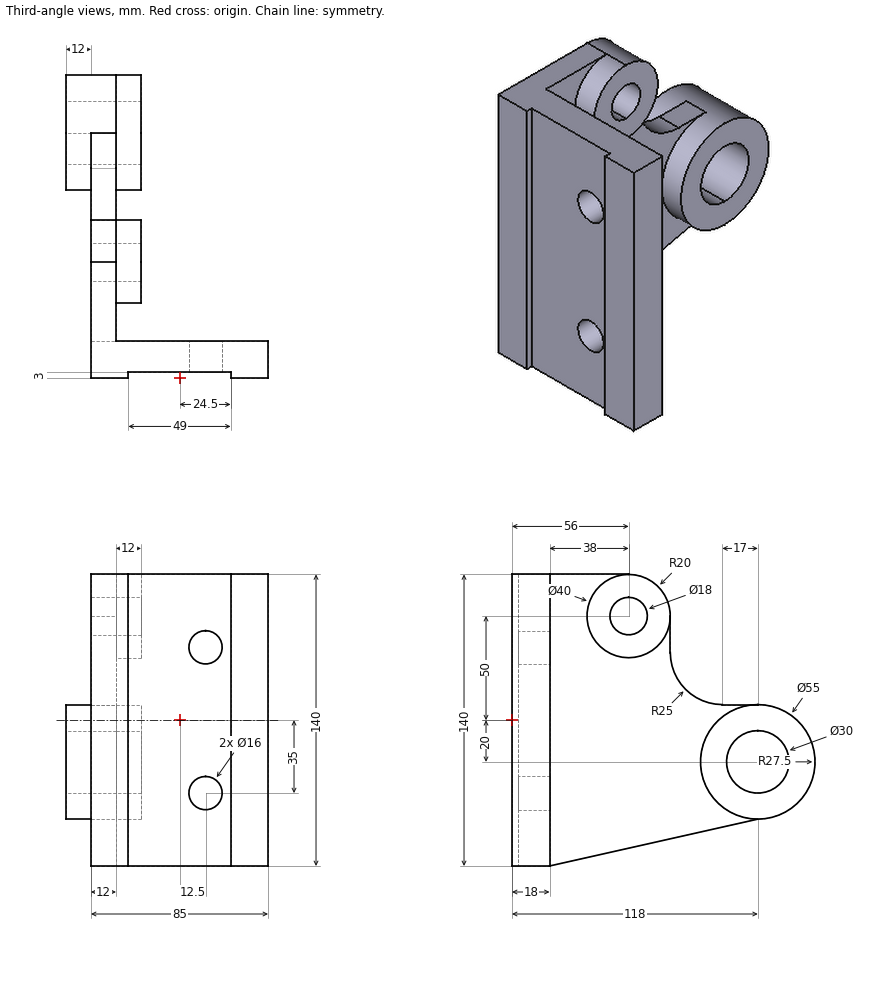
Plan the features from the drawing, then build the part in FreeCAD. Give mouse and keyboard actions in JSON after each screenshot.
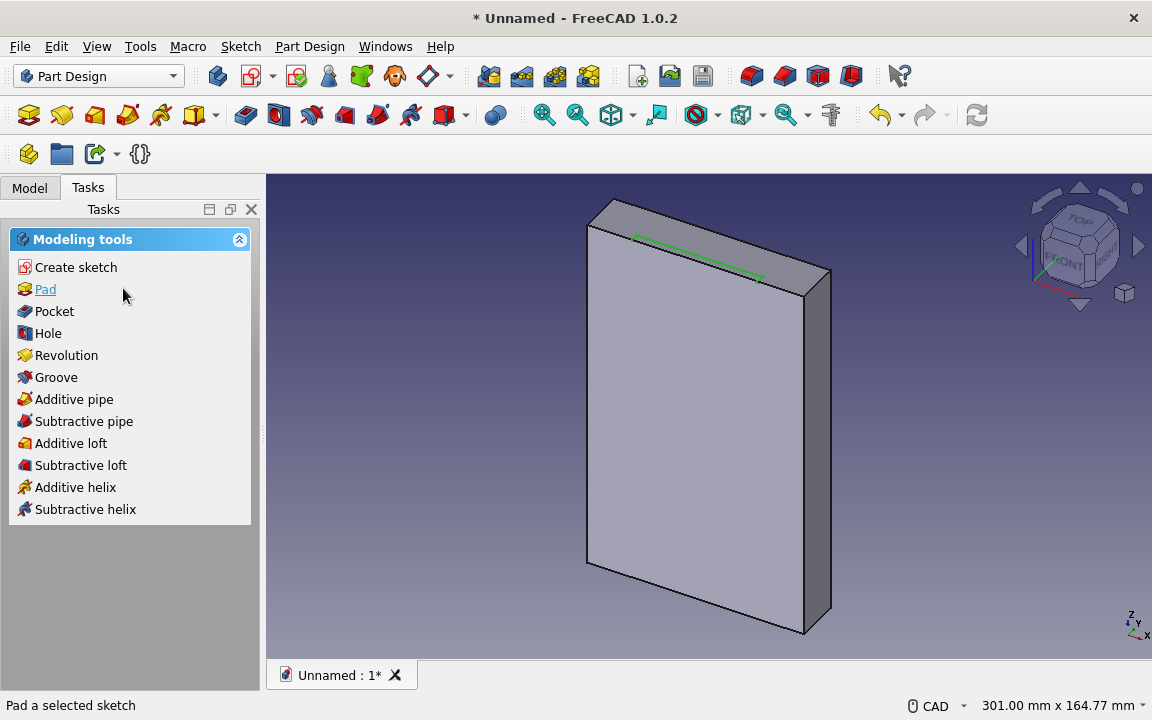
{"action": "left_click", "coordinate": [246, 116]}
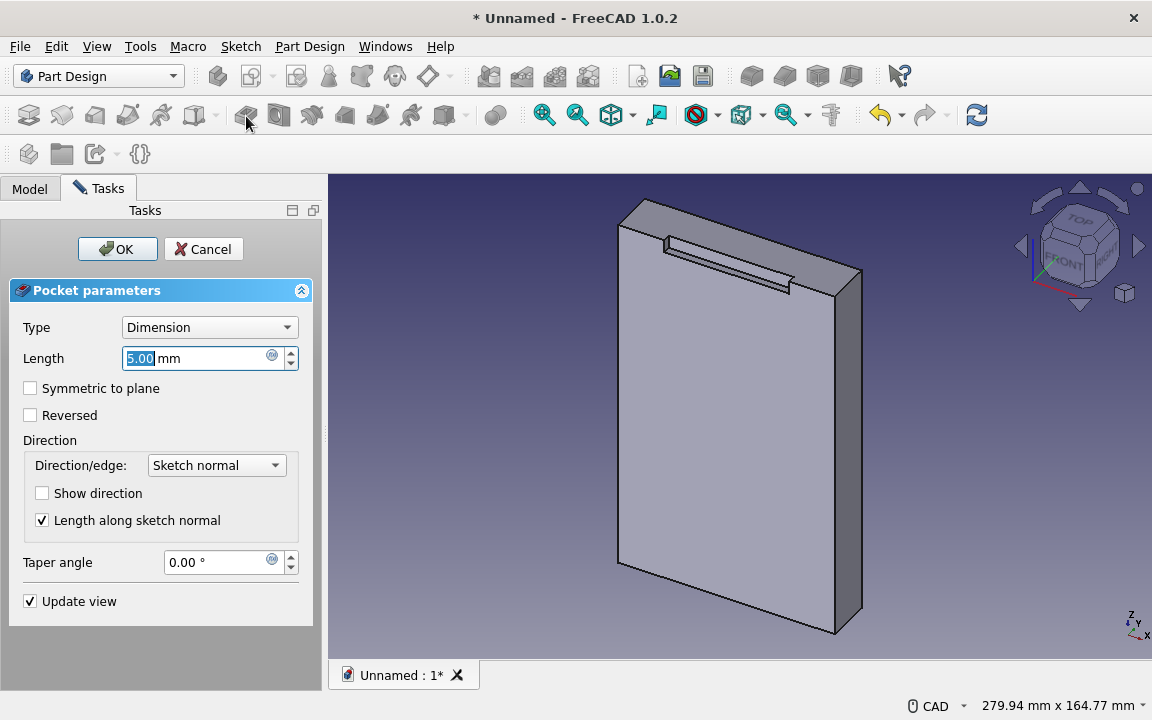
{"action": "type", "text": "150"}
{"action": "key", "text": "Tab"}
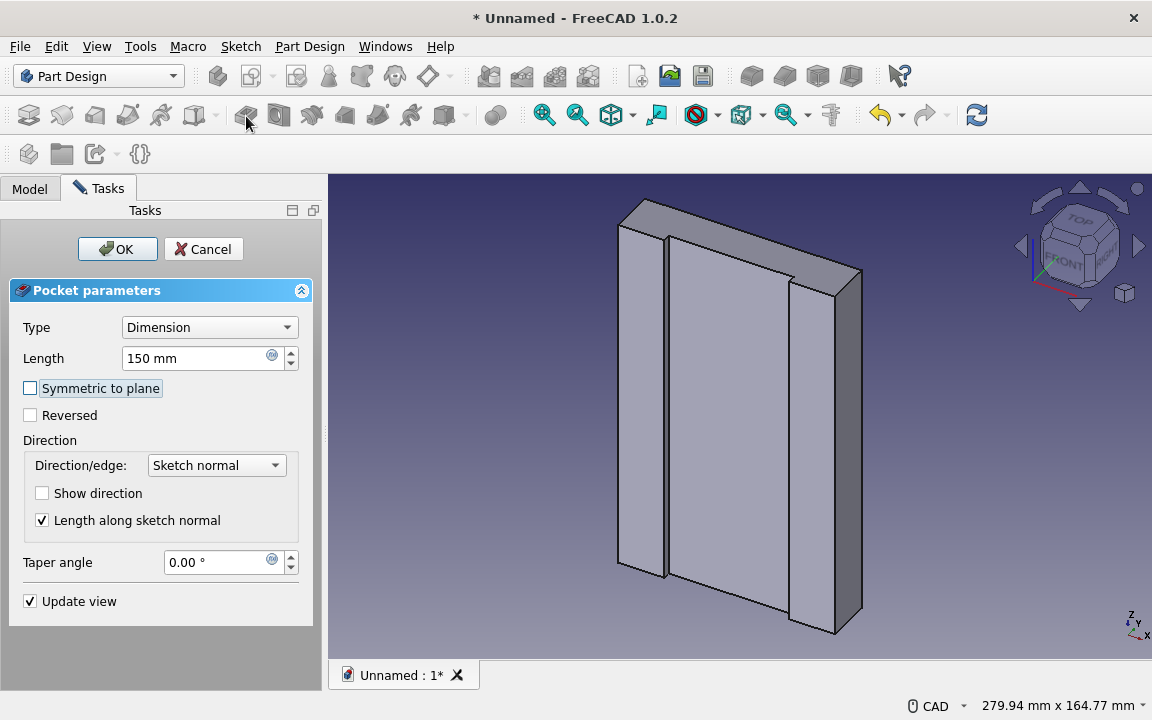
{"action": "left_click", "coordinate": [118, 249]}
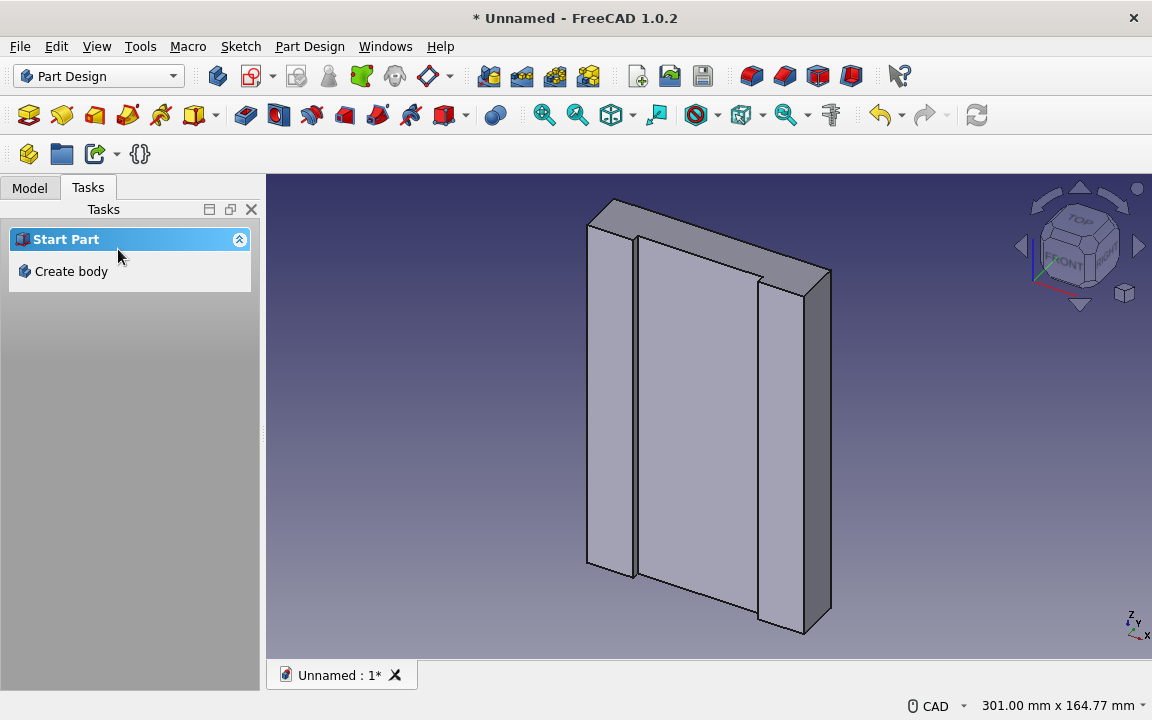
{"action": "key", "text": "6"}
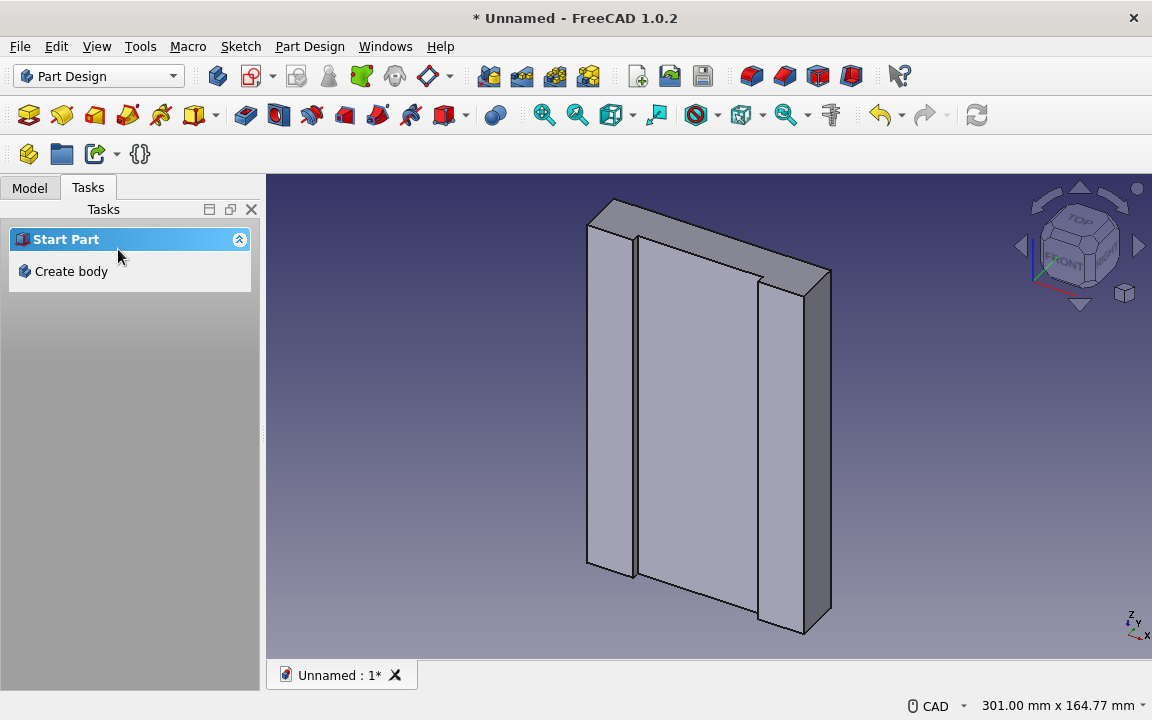
{"action": "left_click", "coordinate": [709, 415]}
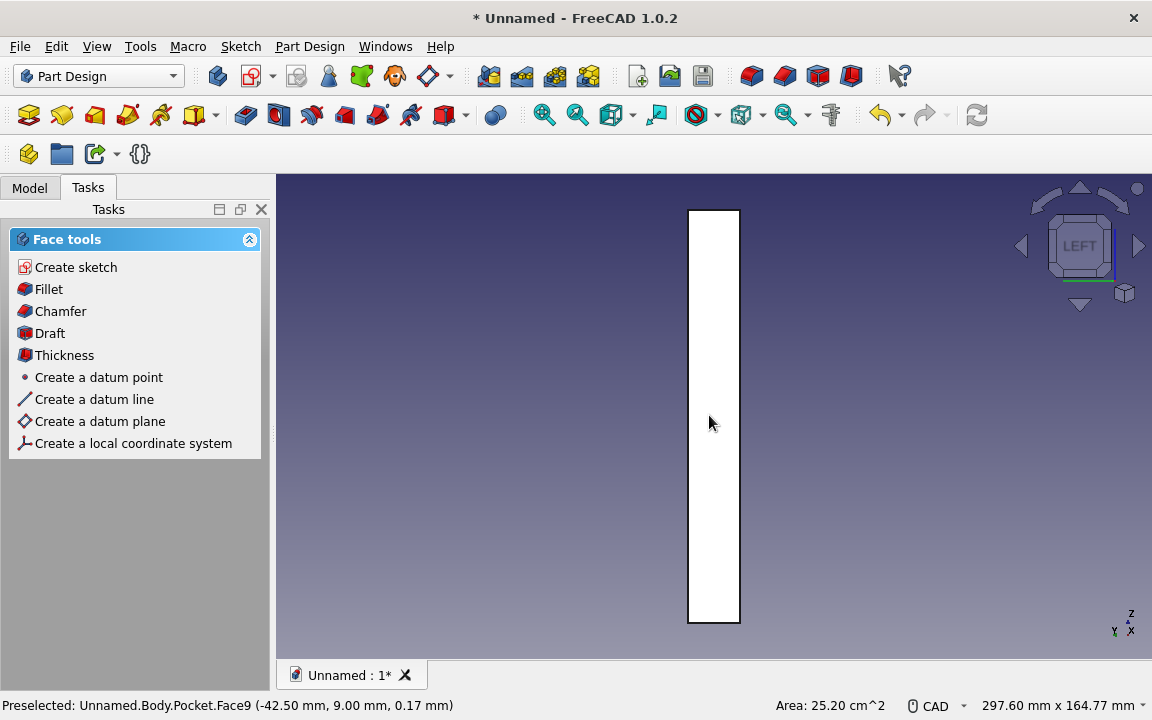
{"action": "left_click", "coordinate": [250, 76]}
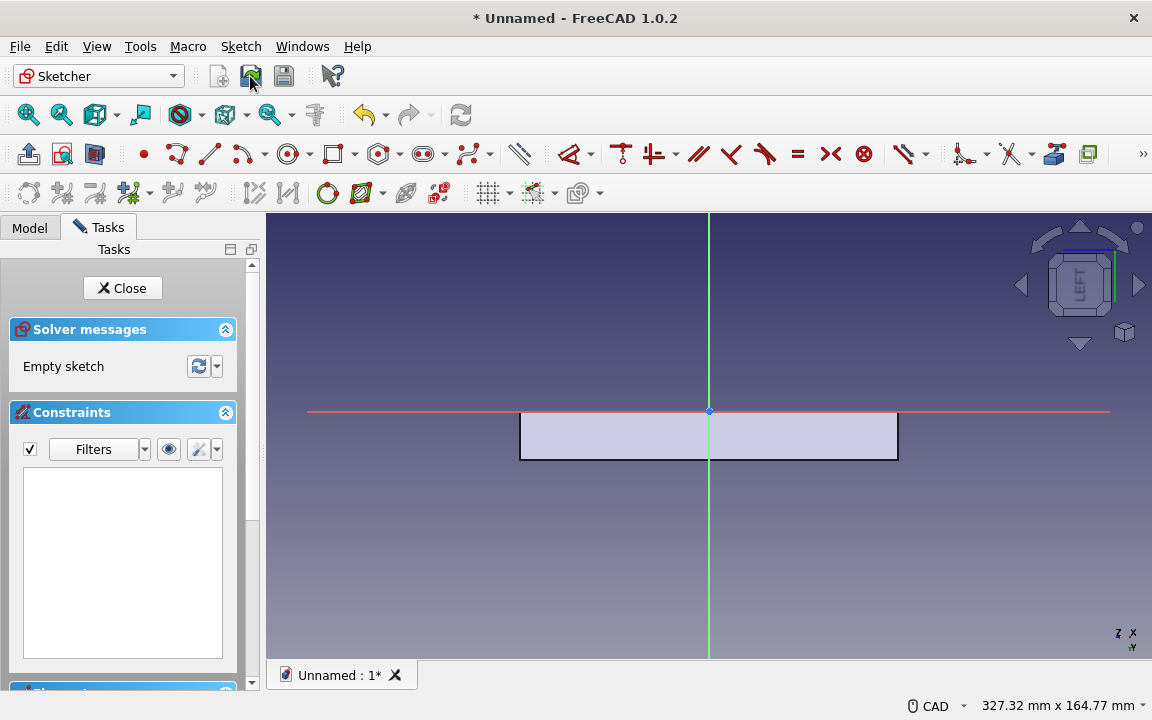
{"action": "scroll", "coordinate": [557, 241], "scroll_direction": "down", "scroll_amount": 3}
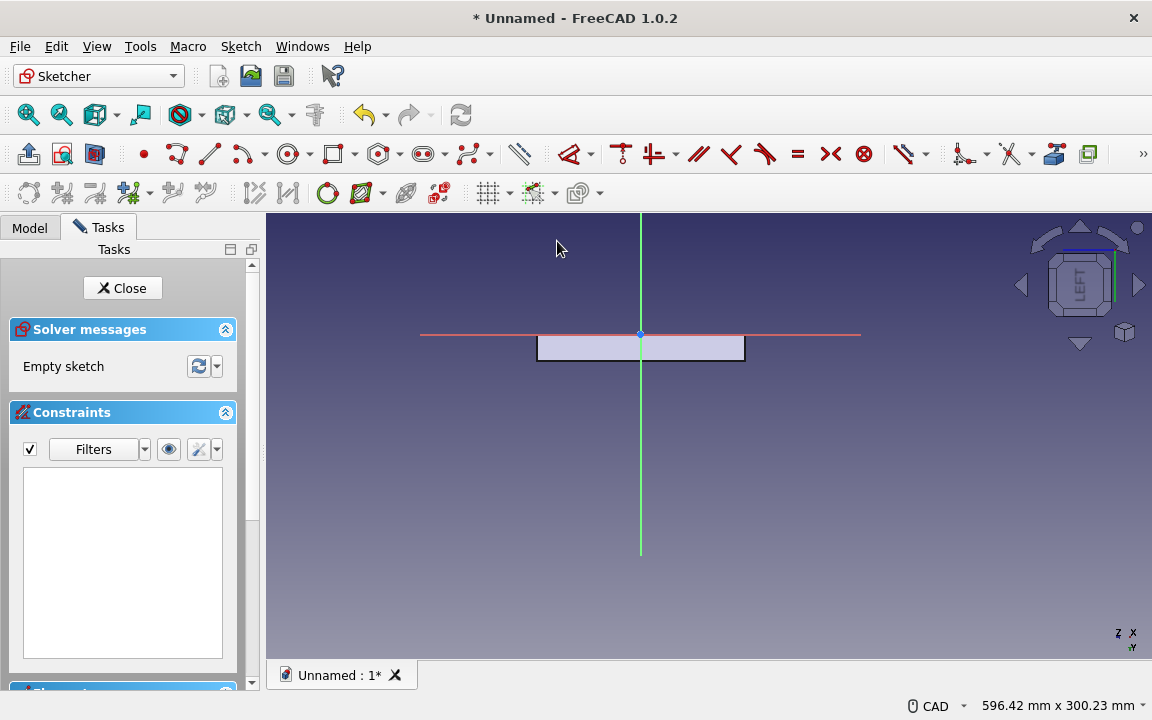
{"action": "left_click", "coordinate": [210, 154]}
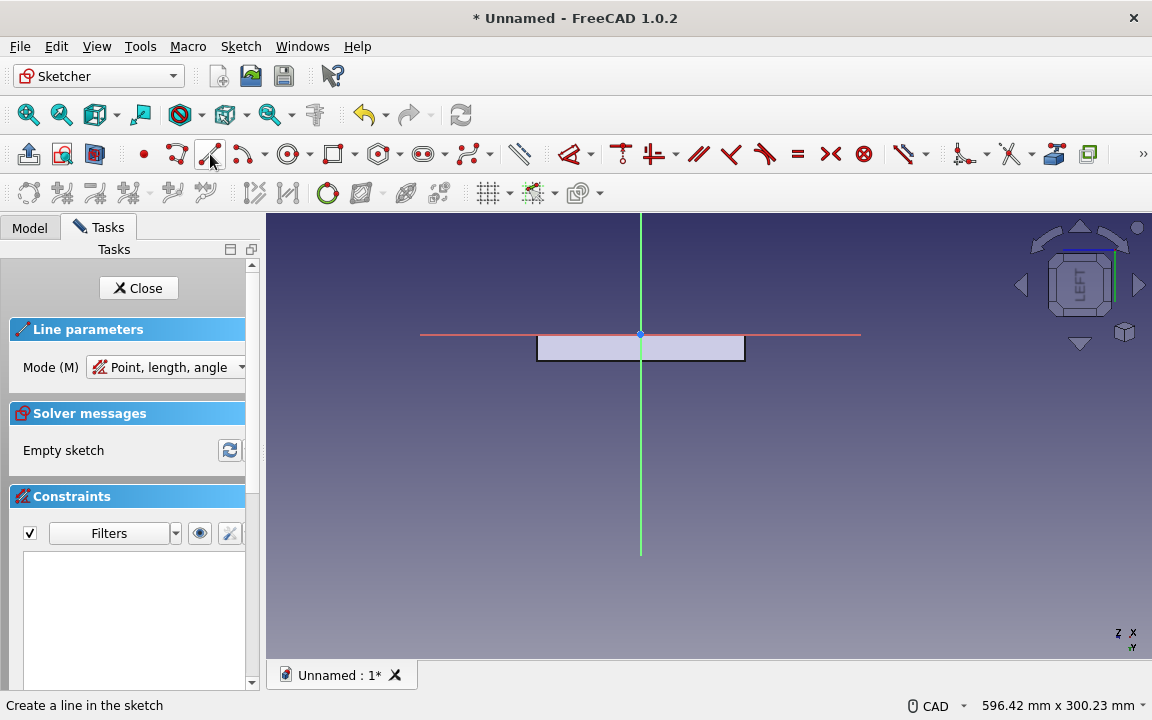
{"action": "left_click", "coordinate": [566, 448]}
{"action": "left_click", "coordinate": [592, 448]}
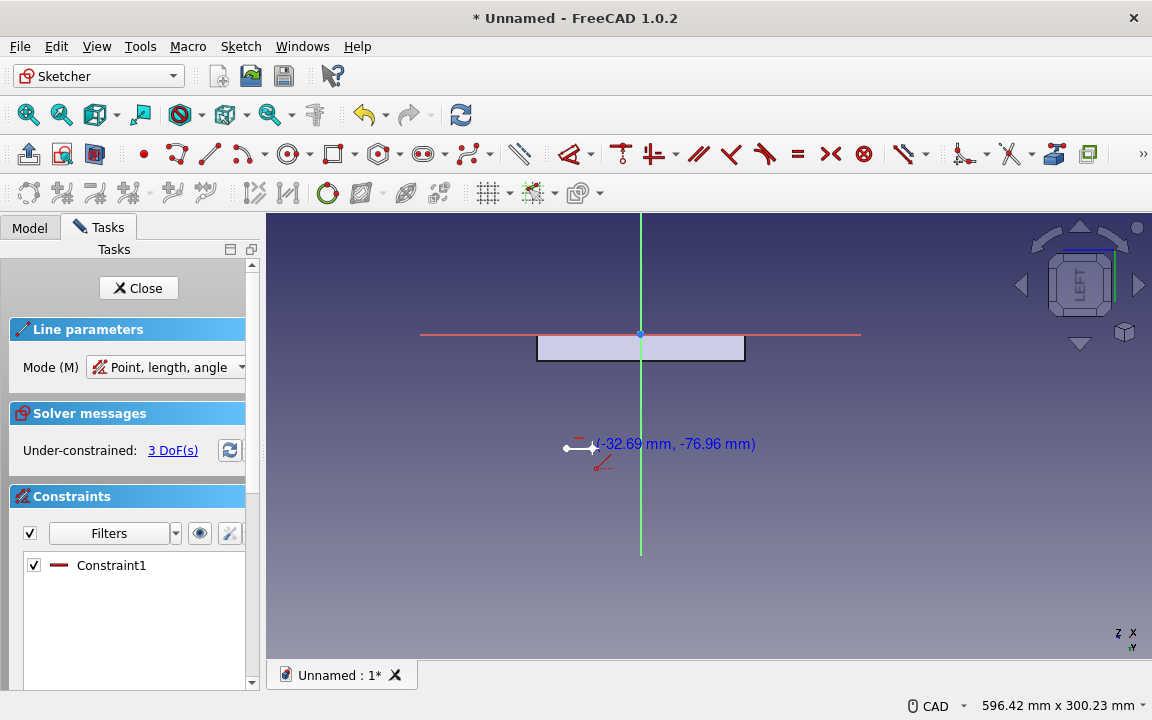
{"action": "scroll", "coordinate": [629, 485], "scroll_direction": "up", "scroll_amount": 2}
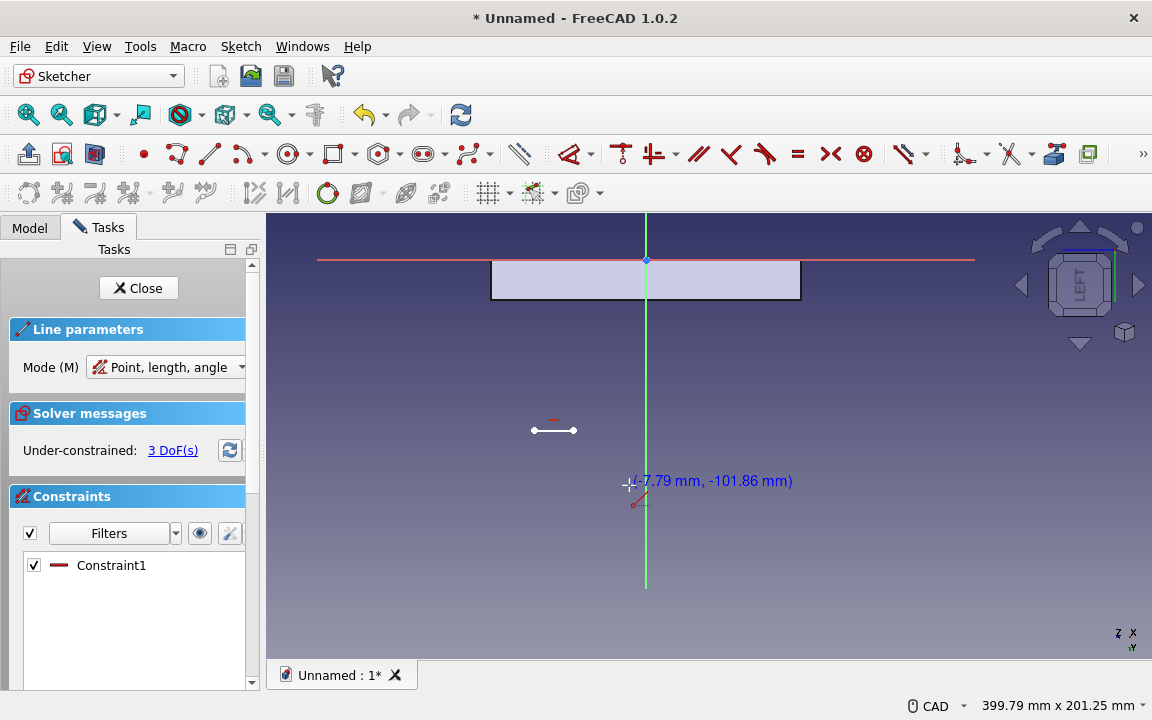
{"action": "left_click", "coordinate": [629, 484]}
{"action": "left_click", "coordinate": [629, 522]}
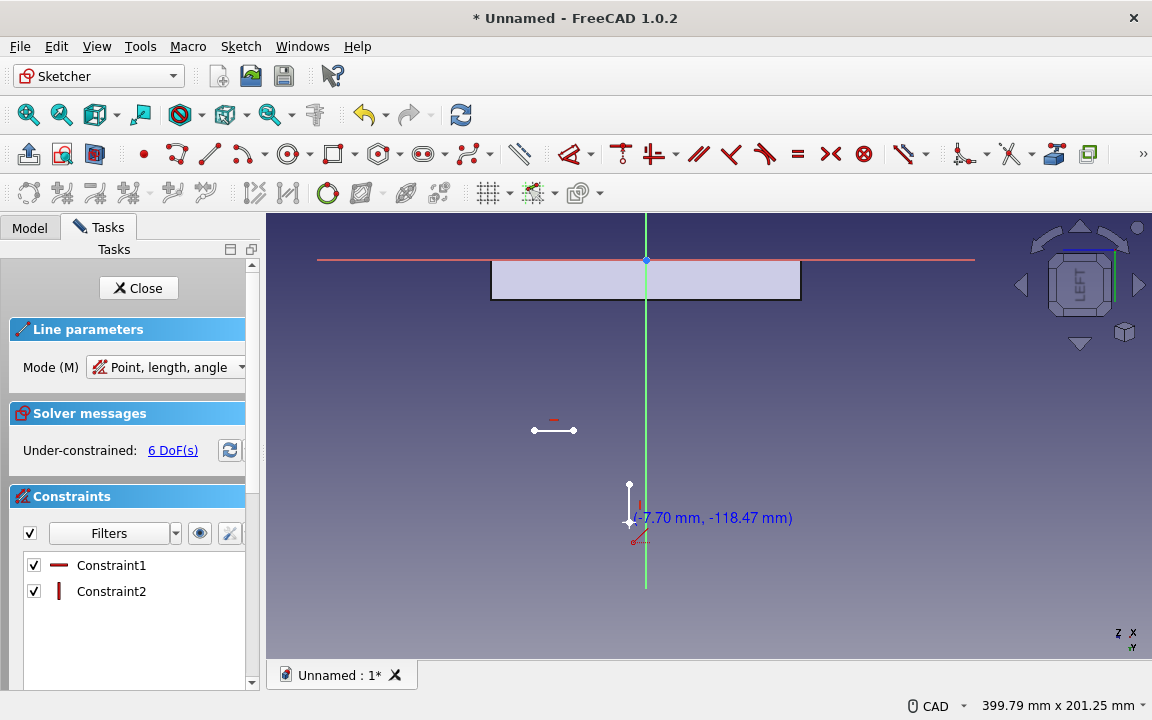
{"action": "left_click", "coordinate": [177, 154]}